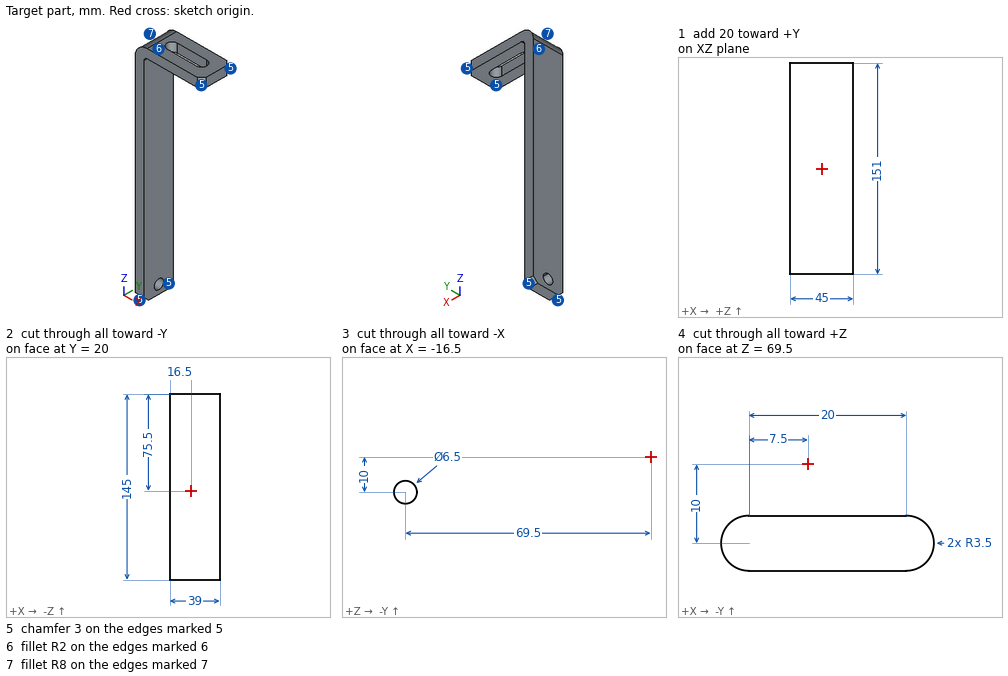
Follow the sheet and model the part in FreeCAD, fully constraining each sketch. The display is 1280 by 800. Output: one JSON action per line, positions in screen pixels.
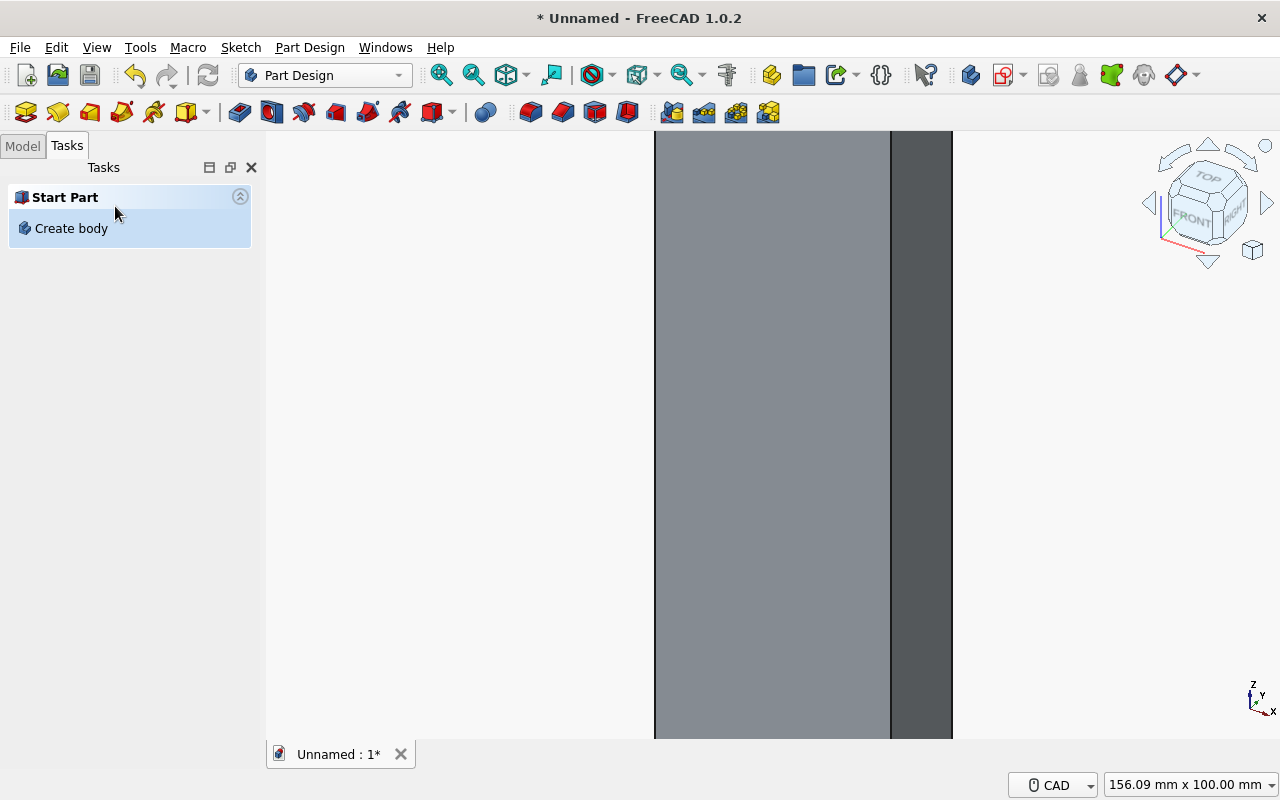
{"action": "left_click", "coordinate": [442, 76]}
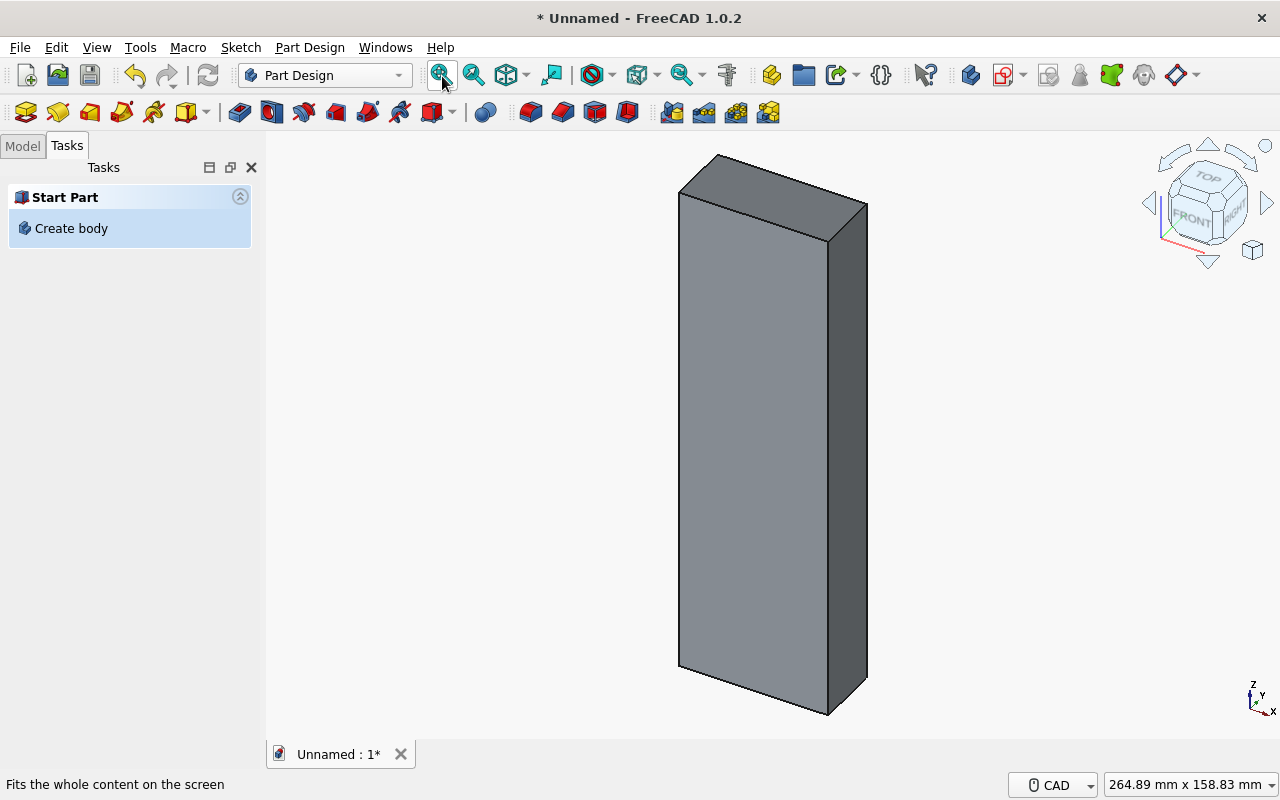
{"action": "key", "text": "4"}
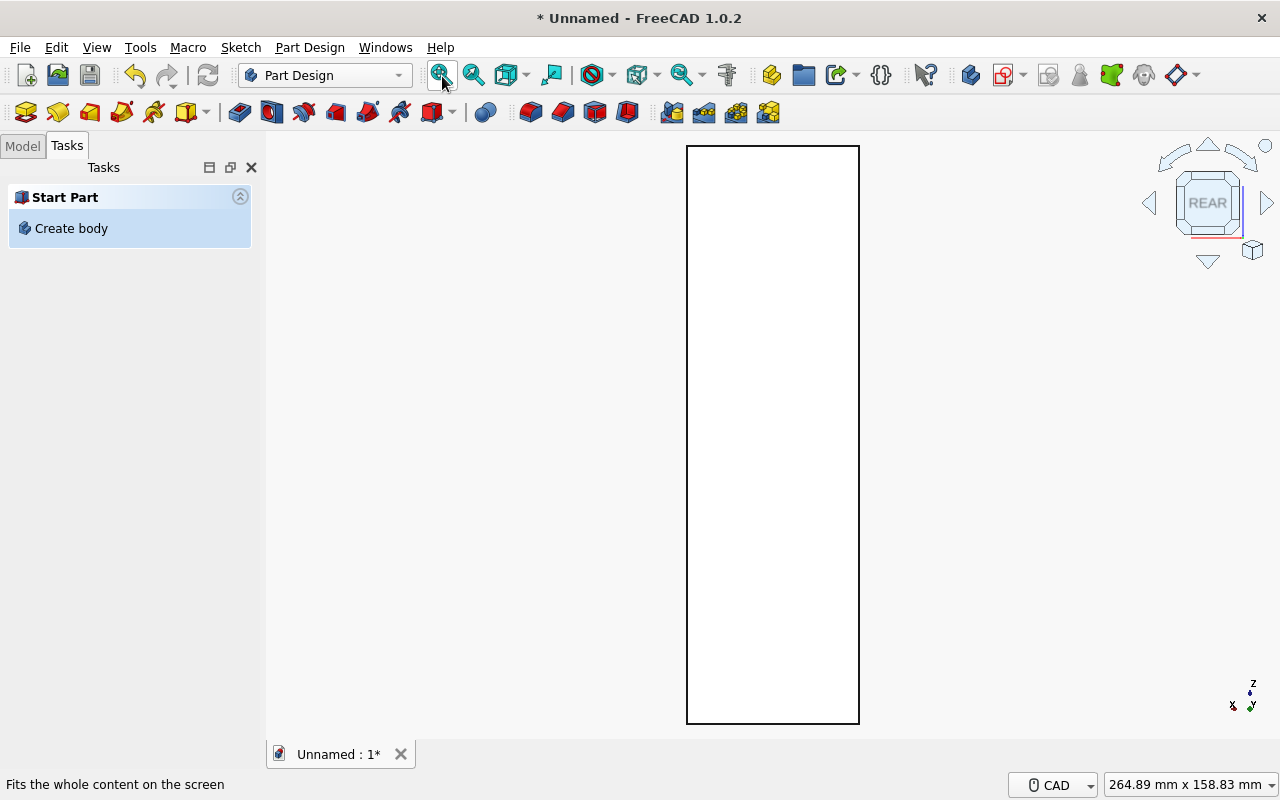
{"action": "left_click", "coordinate": [773, 269]}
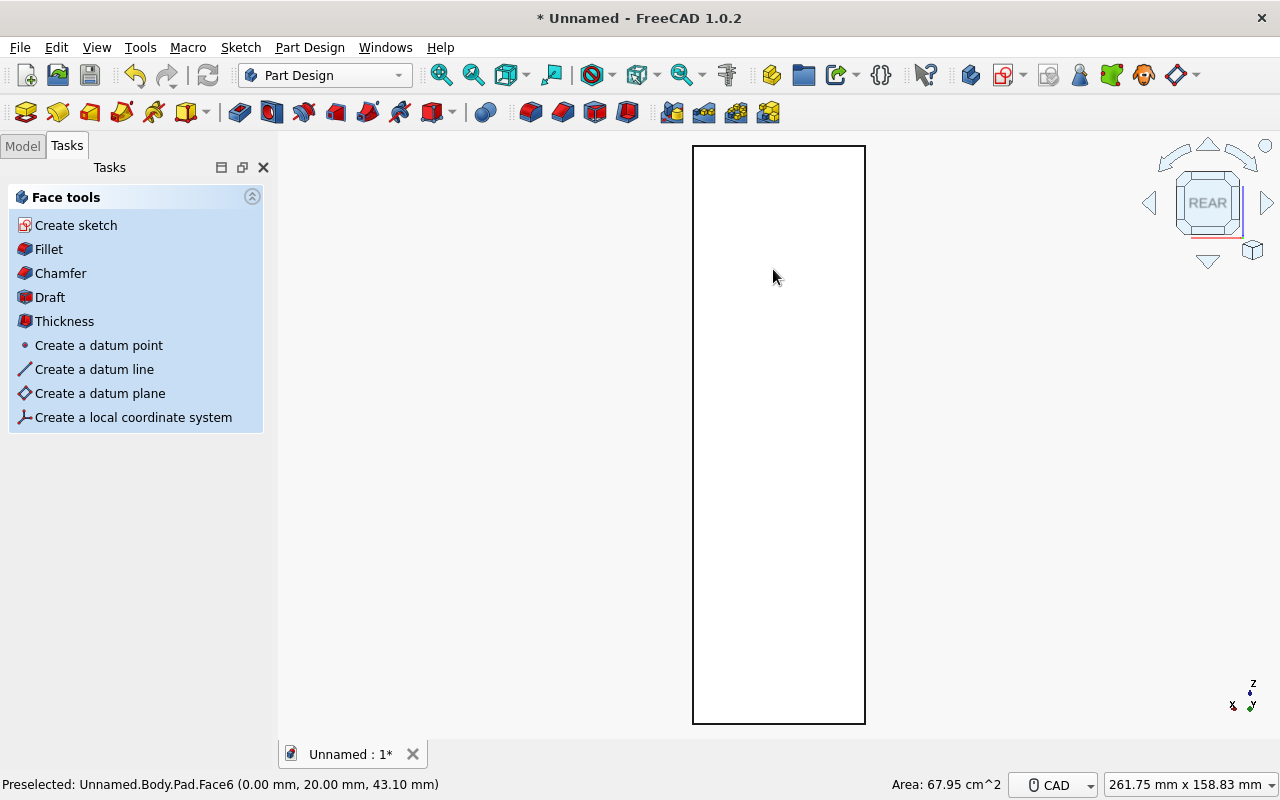
{"action": "left_click", "coordinate": [1004, 76]}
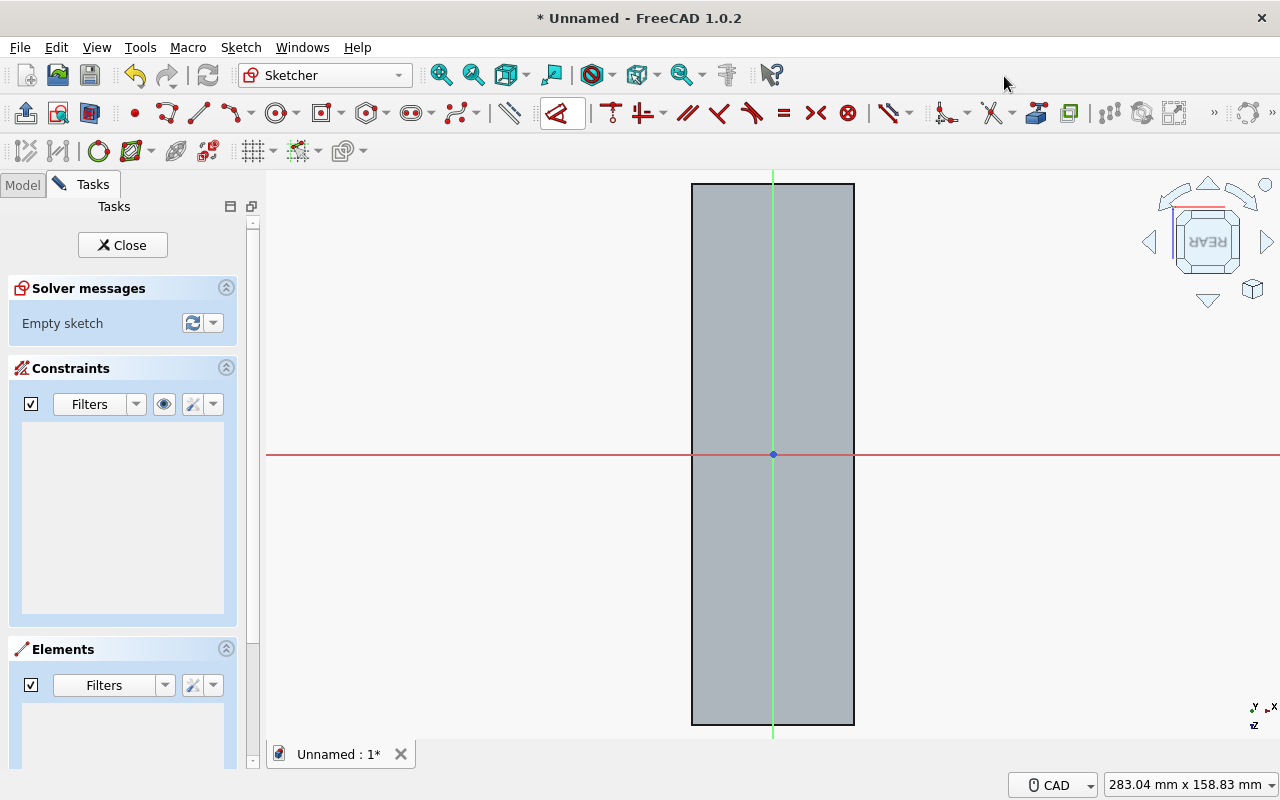
{"action": "scroll", "coordinate": [543, 476], "scroll_direction": "down", "scroll_amount": 2}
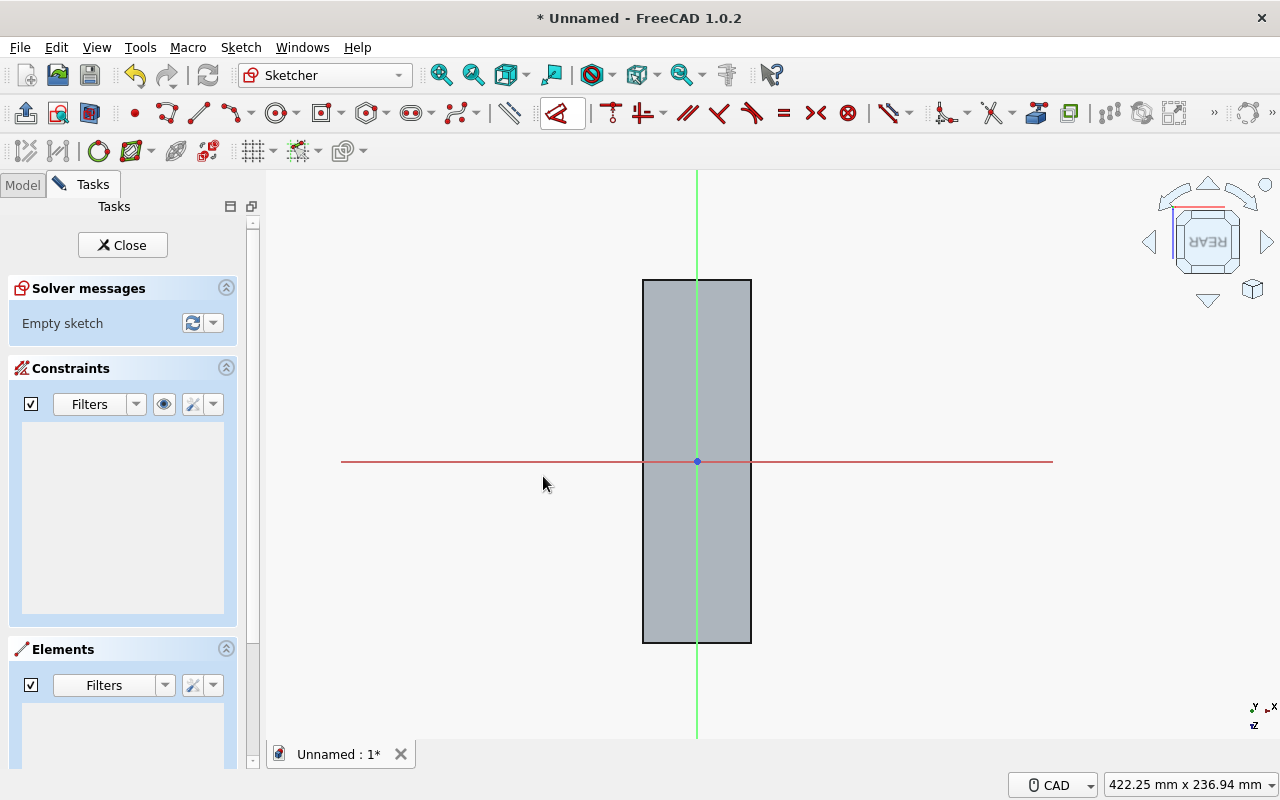
{"action": "left_click", "coordinate": [344, 114]}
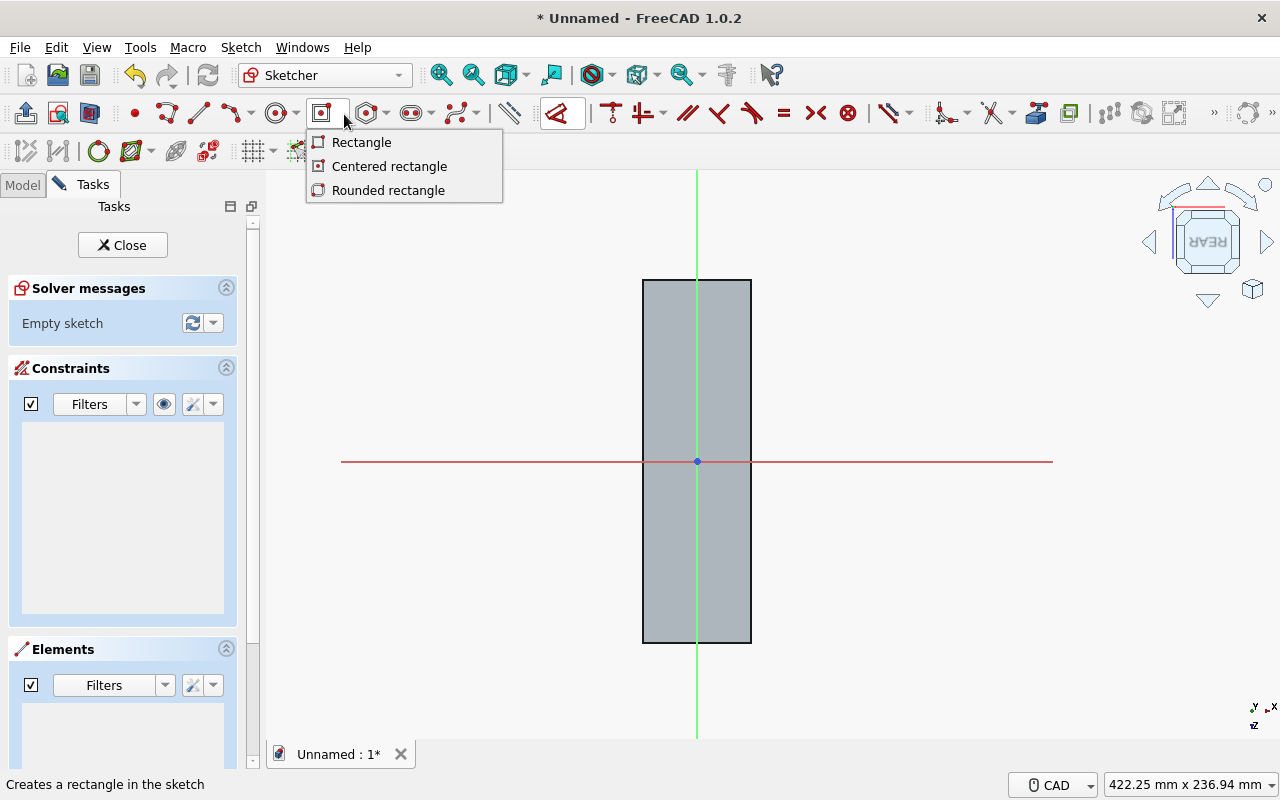
{"action": "left_click", "coordinate": [404, 142]}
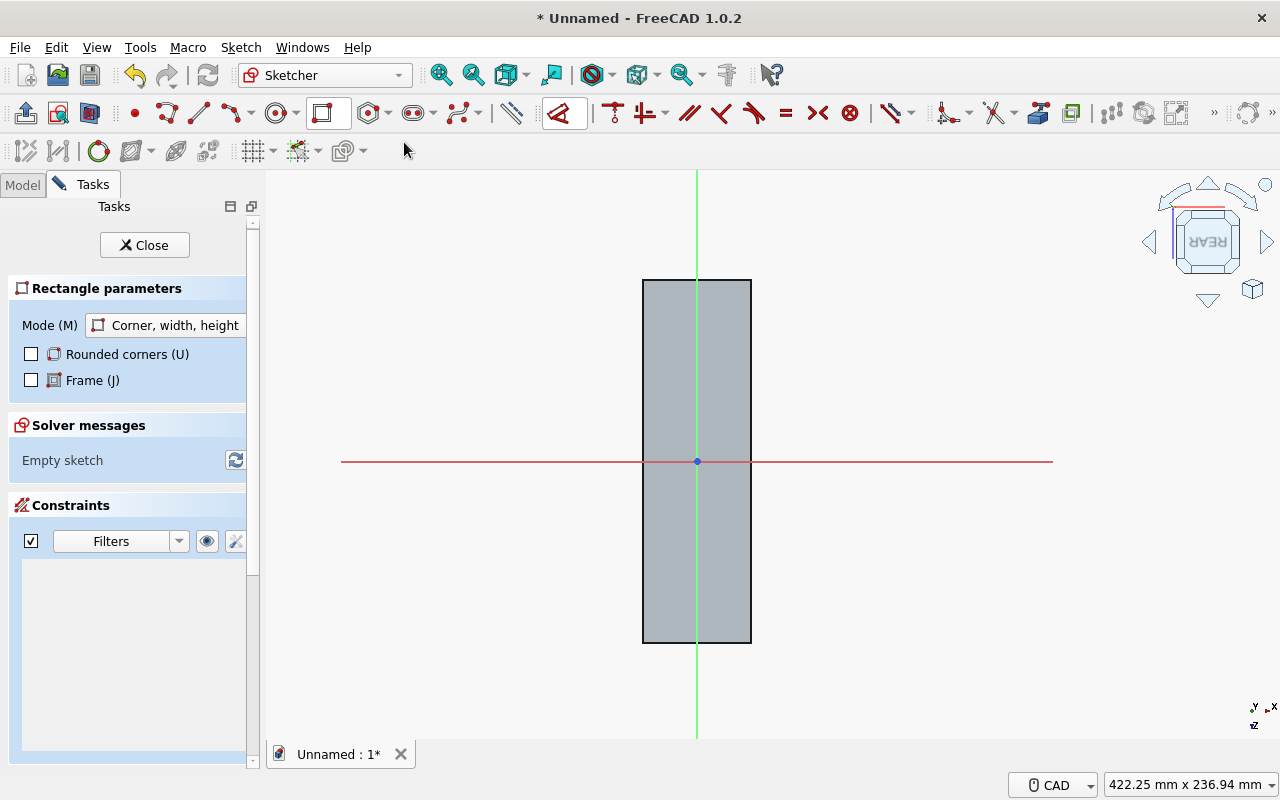
{"action": "left_click", "coordinate": [658, 280]}
{"action": "left_click", "coordinate": [751, 629]}
{"action": "key", "text": "Escape"}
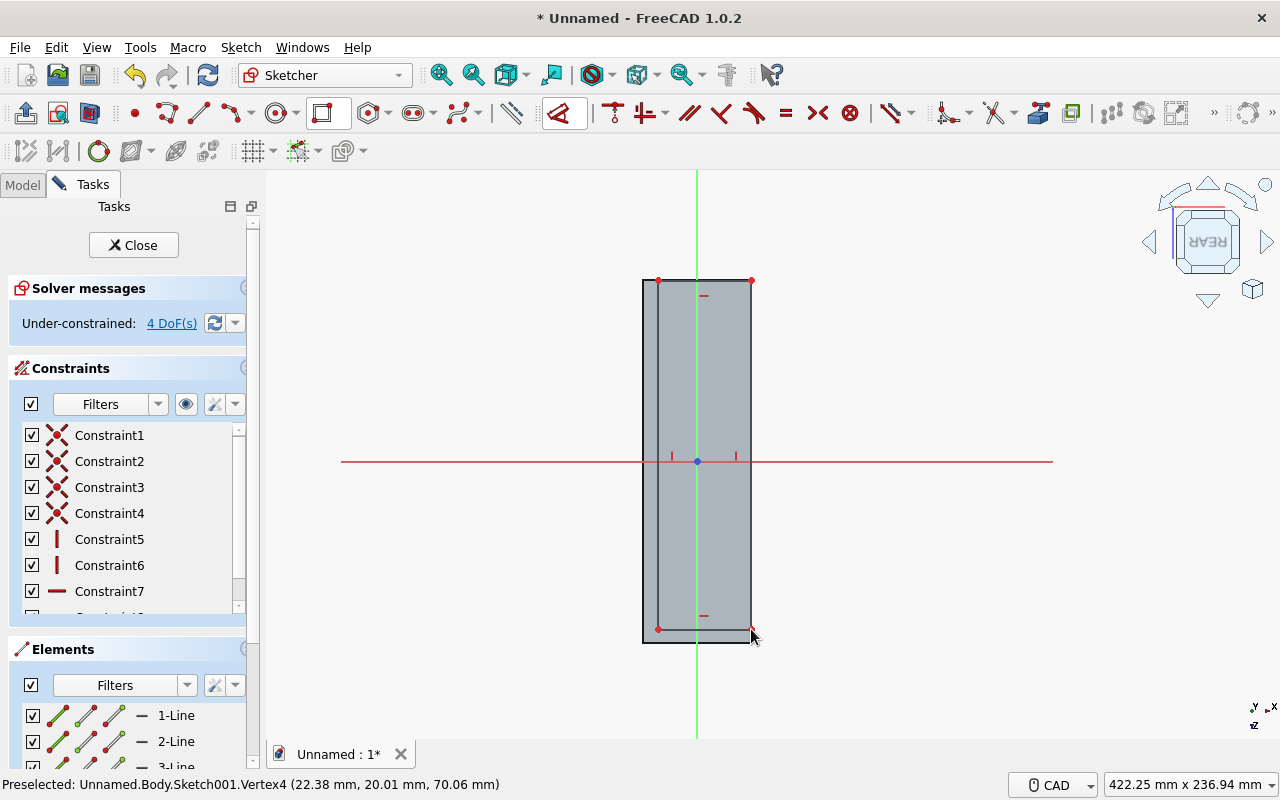
{"action": "left_click", "coordinate": [686, 630]}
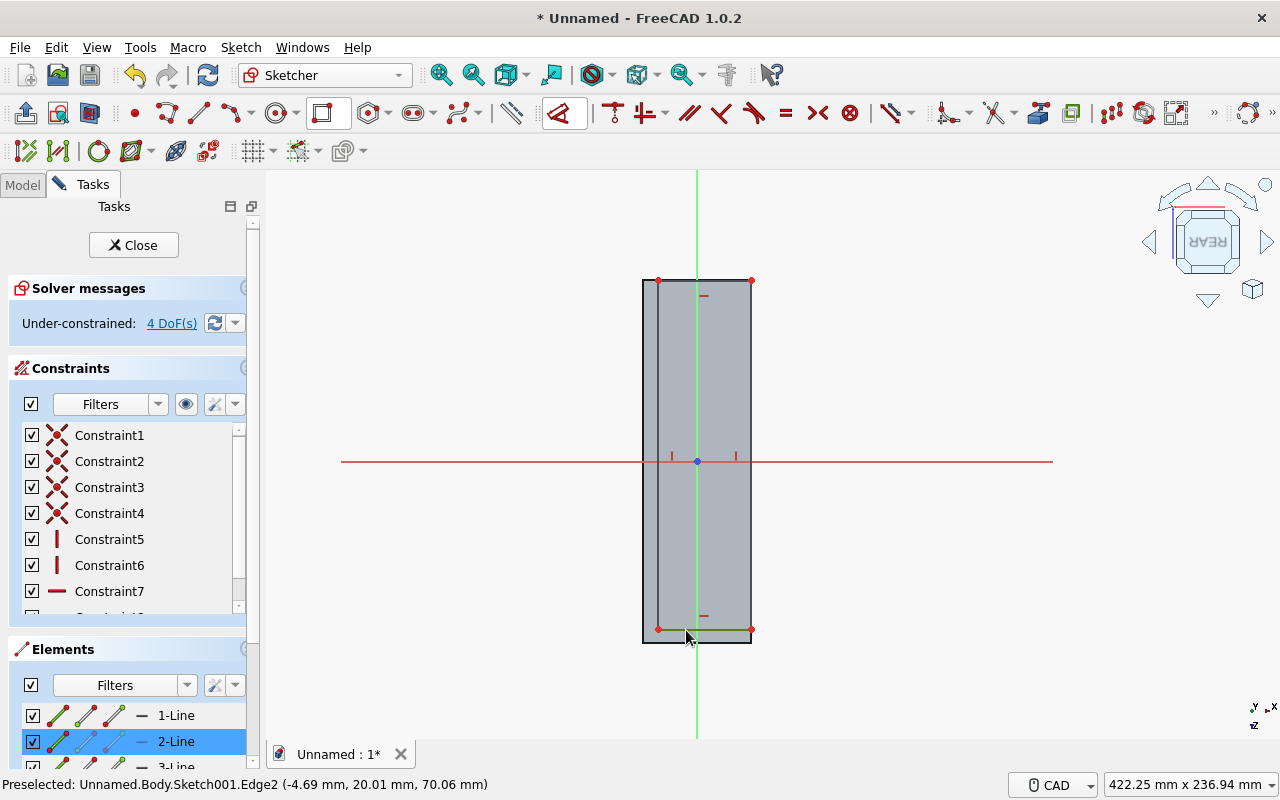
{"action": "key", "text": "l"}